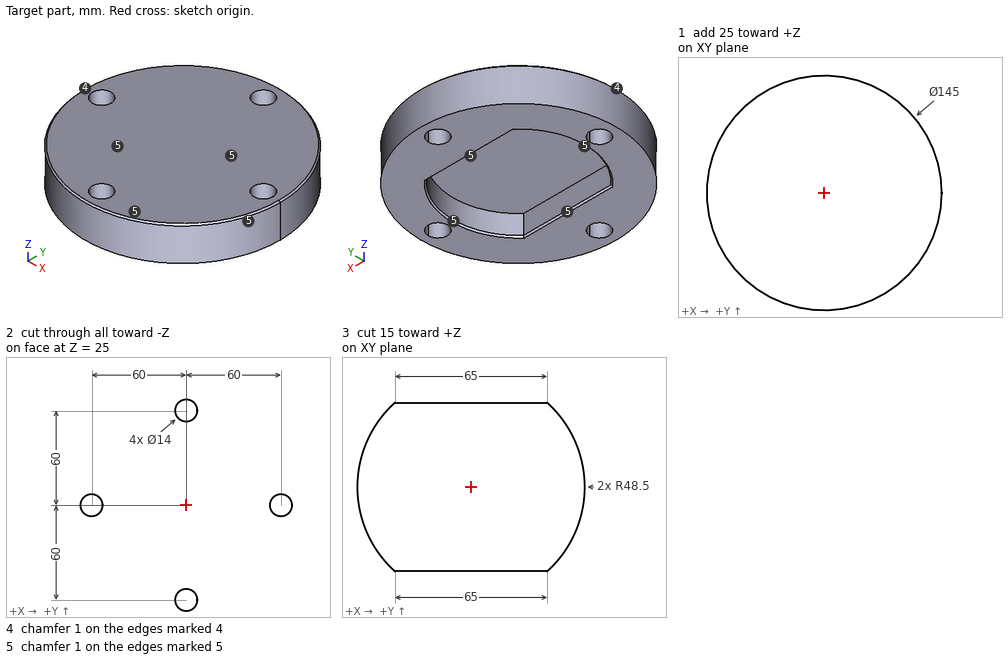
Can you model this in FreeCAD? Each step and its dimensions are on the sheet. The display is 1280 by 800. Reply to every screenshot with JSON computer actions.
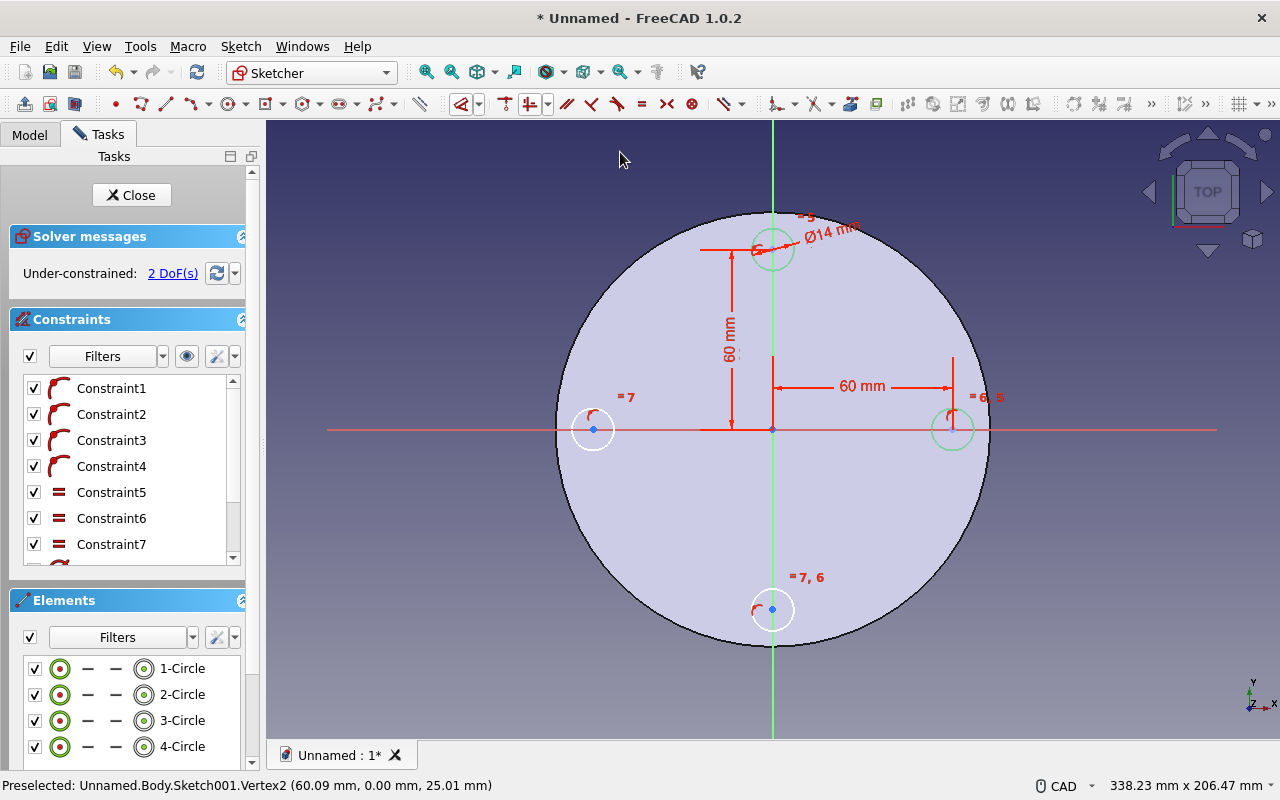
{"action": "left_click", "coordinate": [773, 610]}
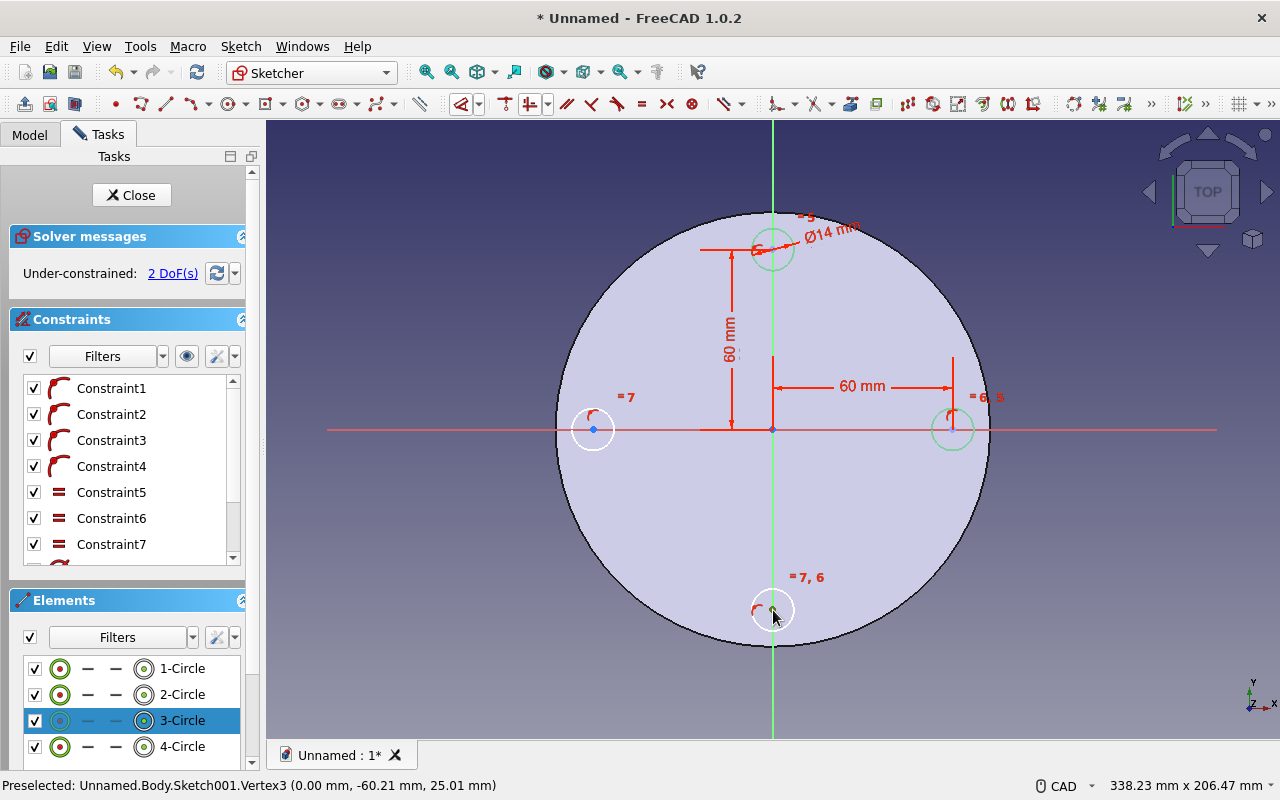
{"action": "key", "text": "i"}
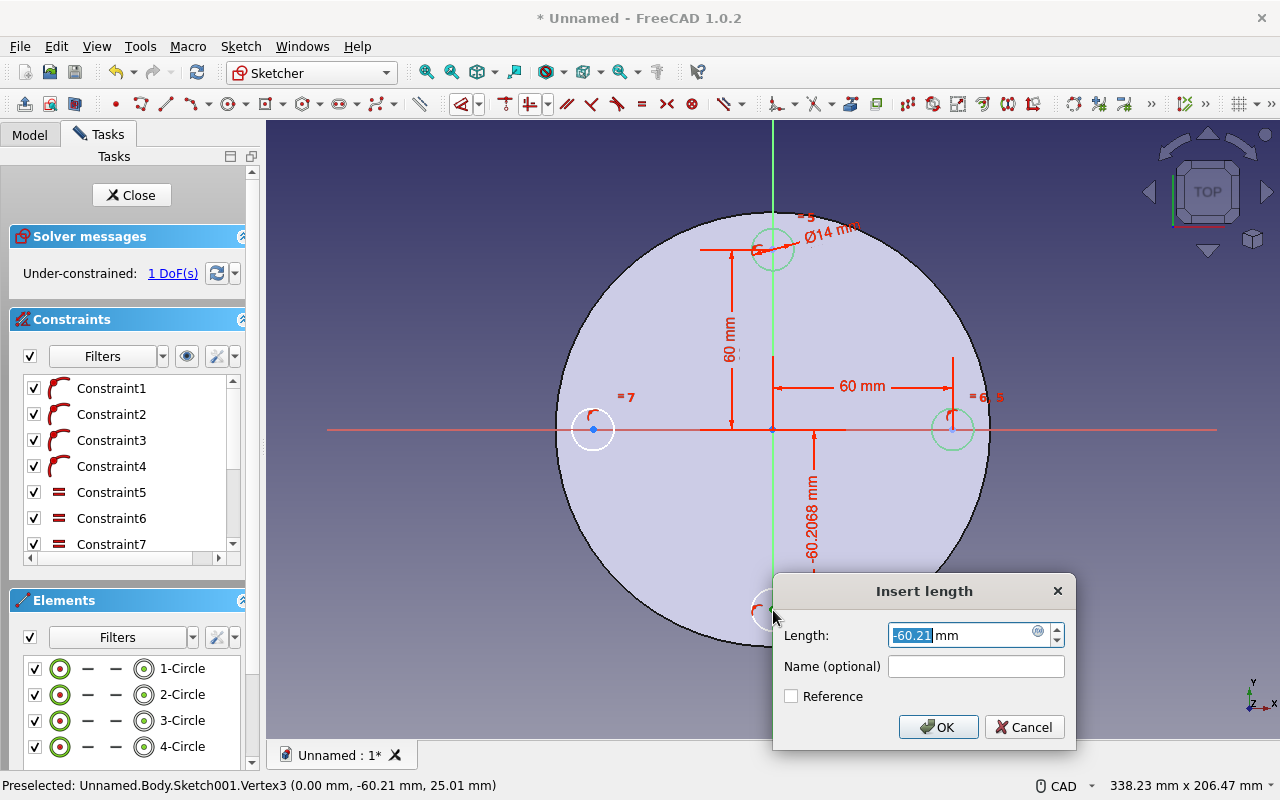
{"action": "type", "text": "-60"}
{"action": "key", "text": "Return"}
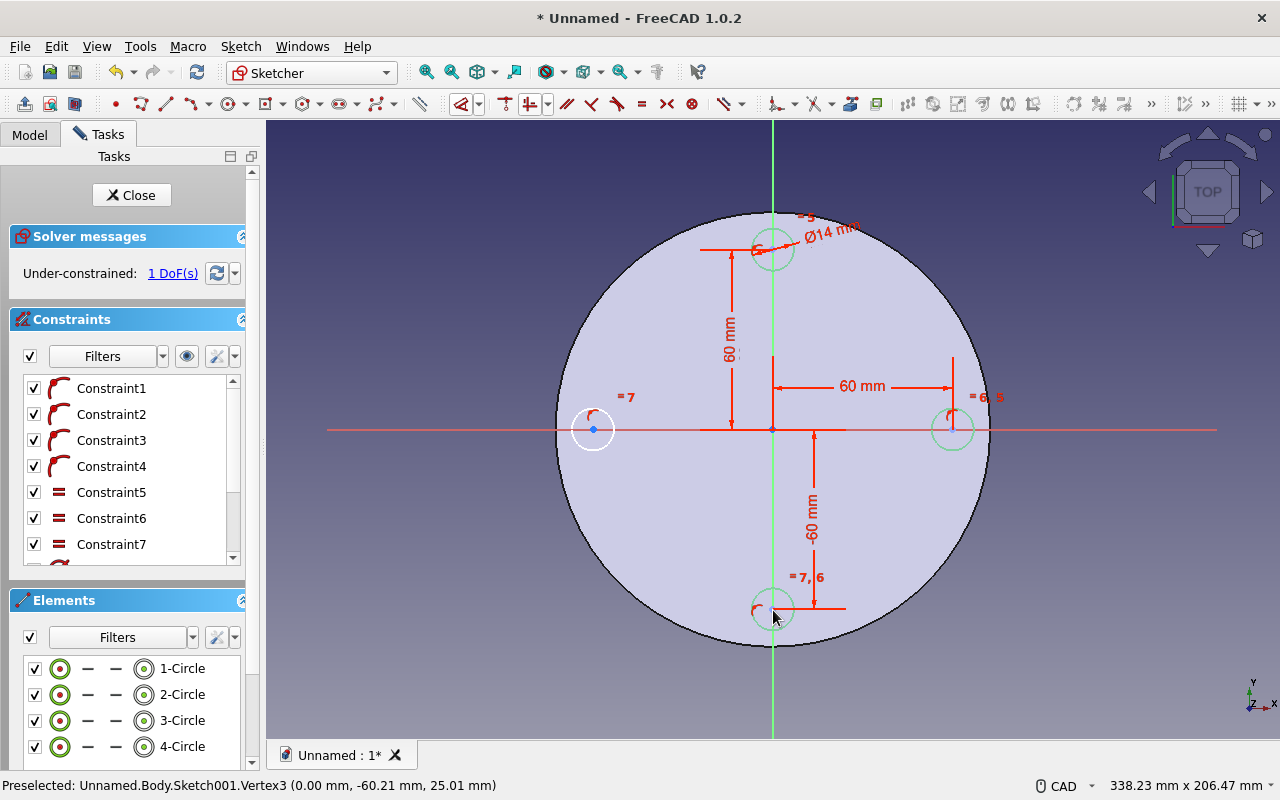
{"action": "left_click", "coordinate": [593, 430]}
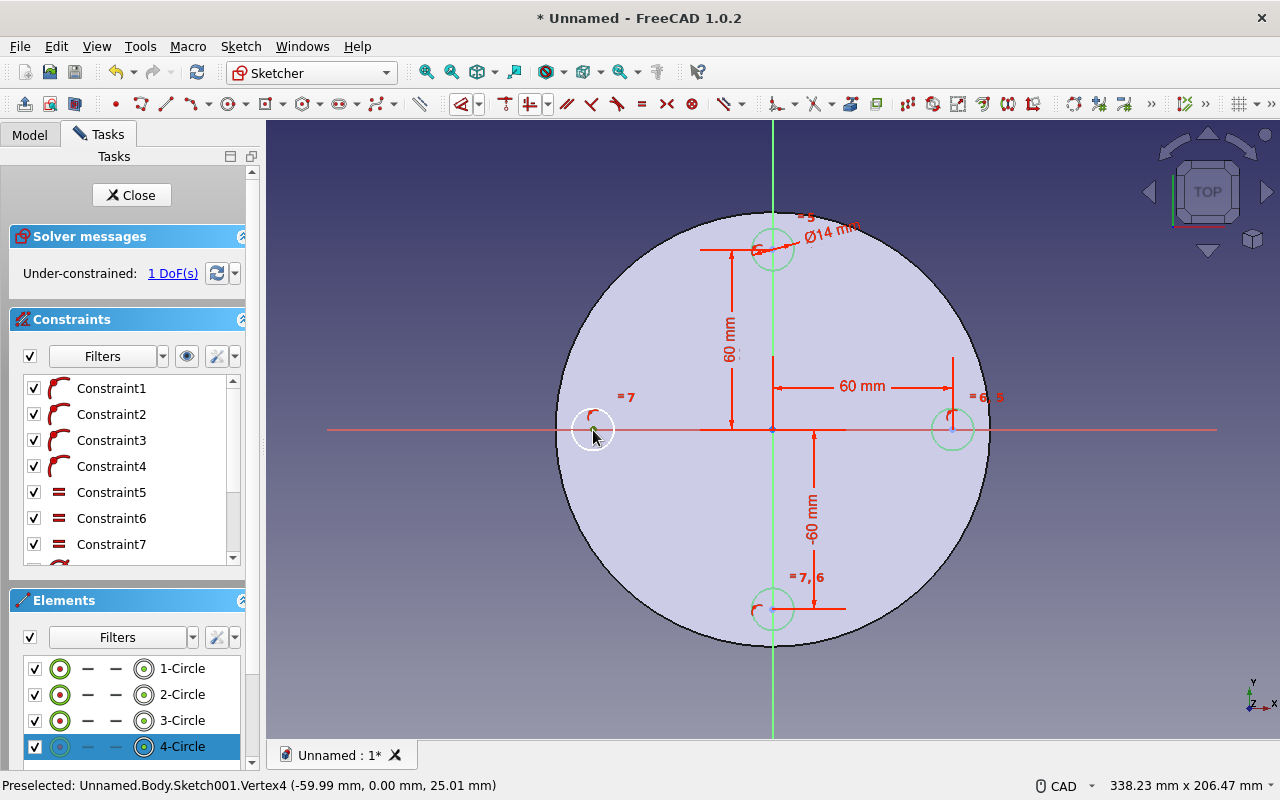
{"action": "left_click", "coordinate": [478, 104]}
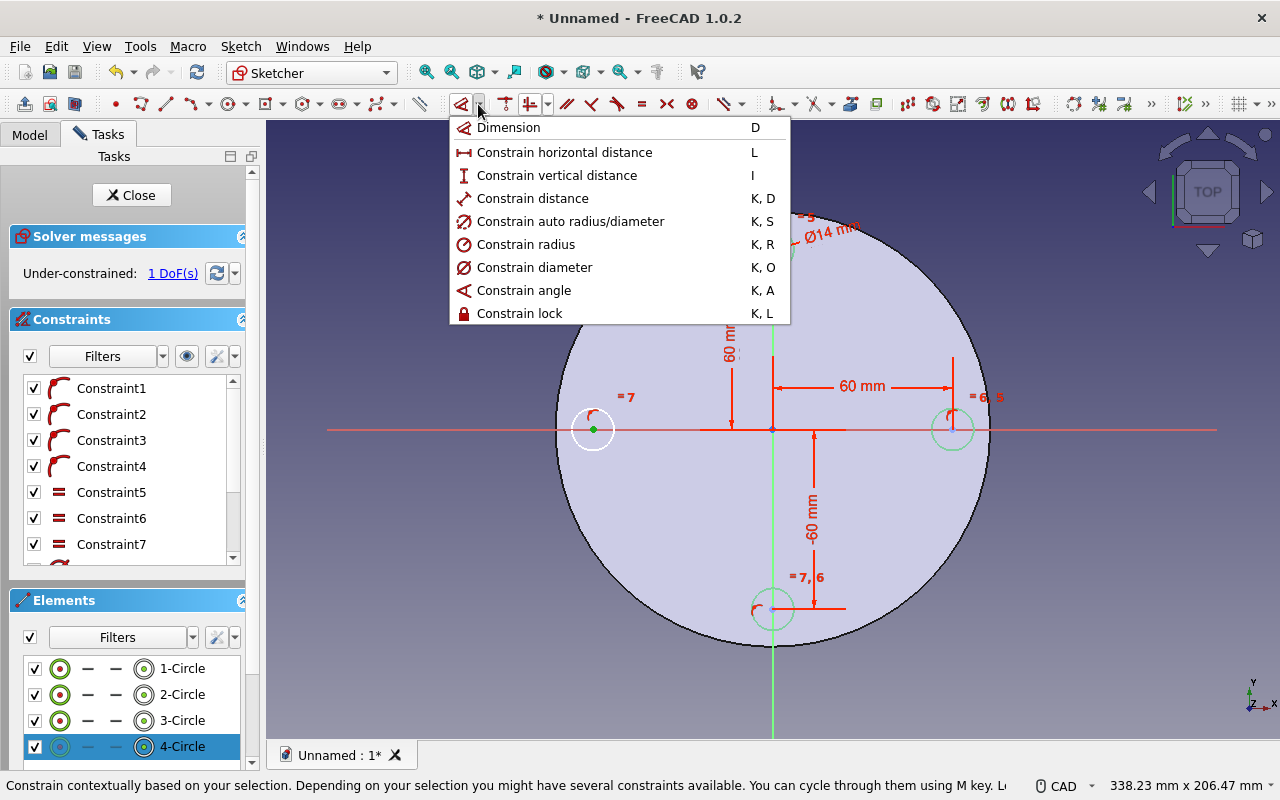
{"action": "left_click", "coordinate": [620, 152]}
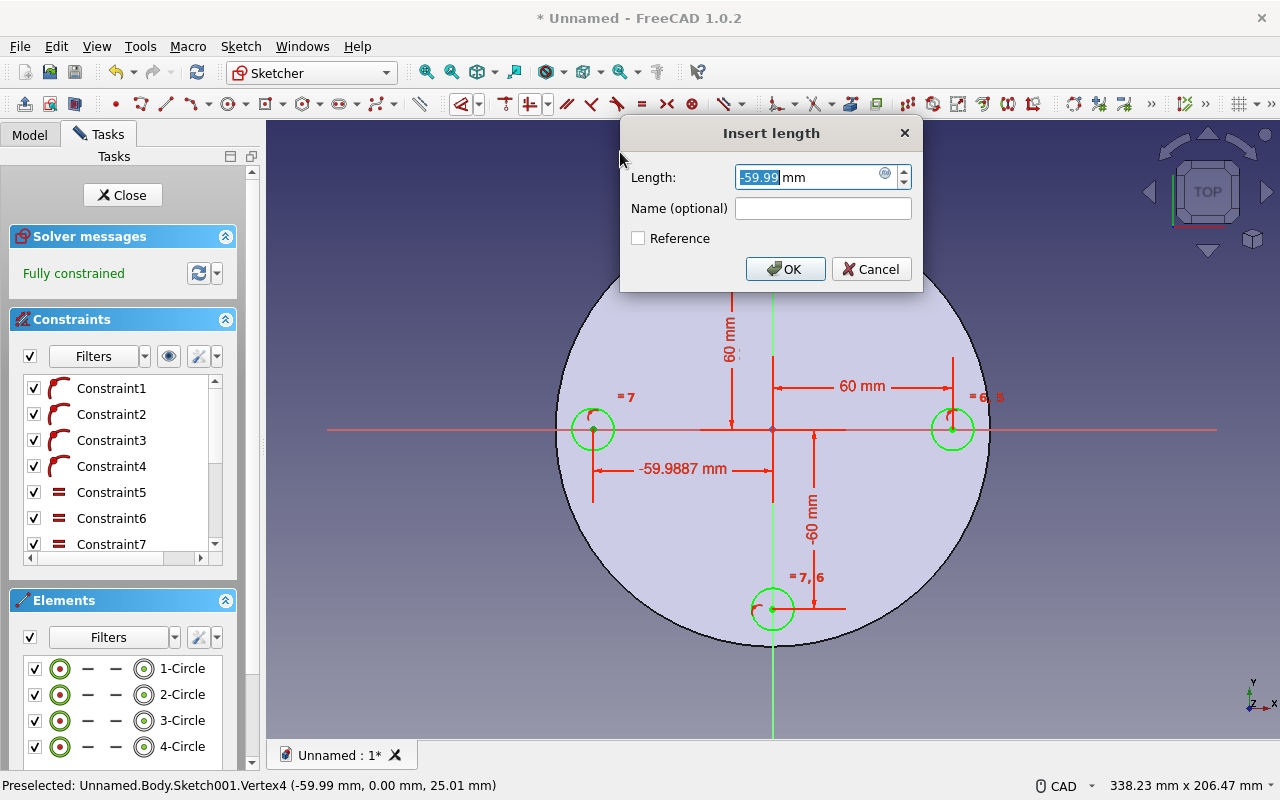
{"action": "type", "text": "-60"}
{"action": "key", "text": "Return"}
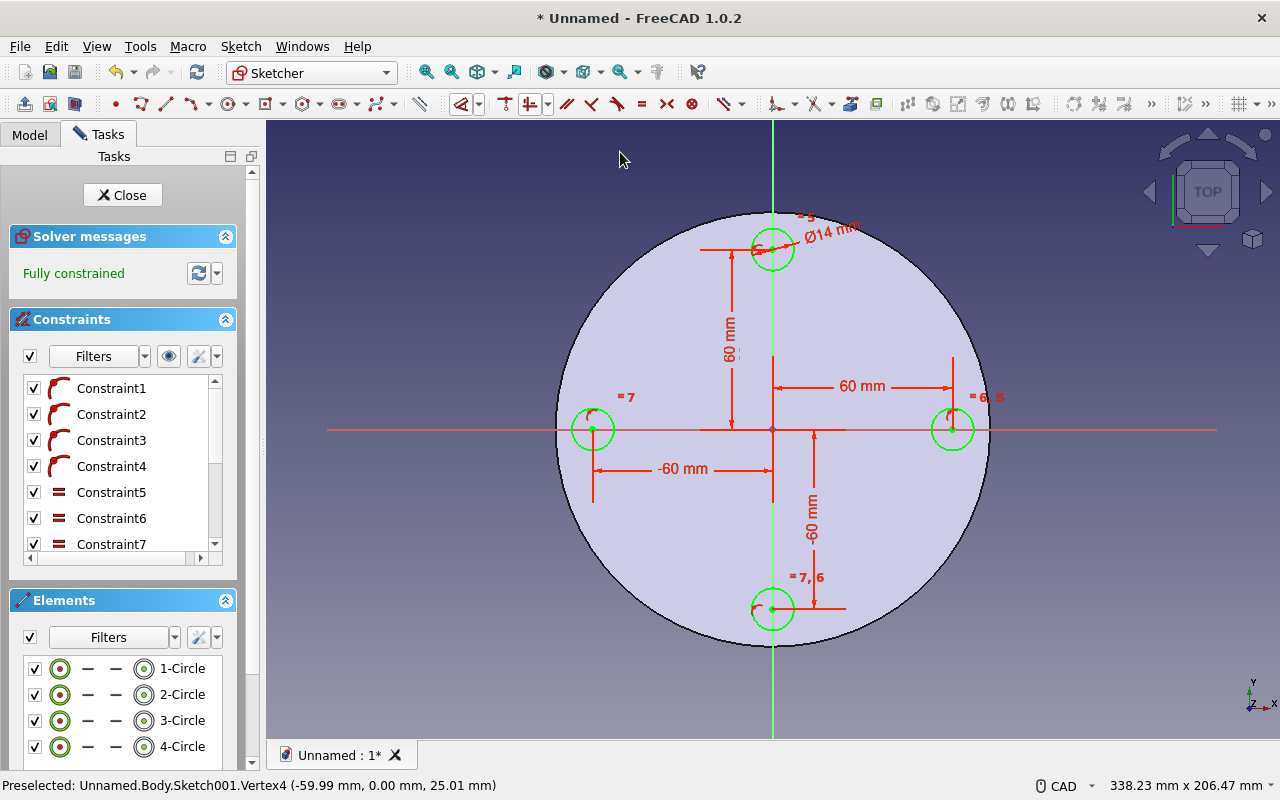
{"action": "left_click", "coordinate": [123, 195]}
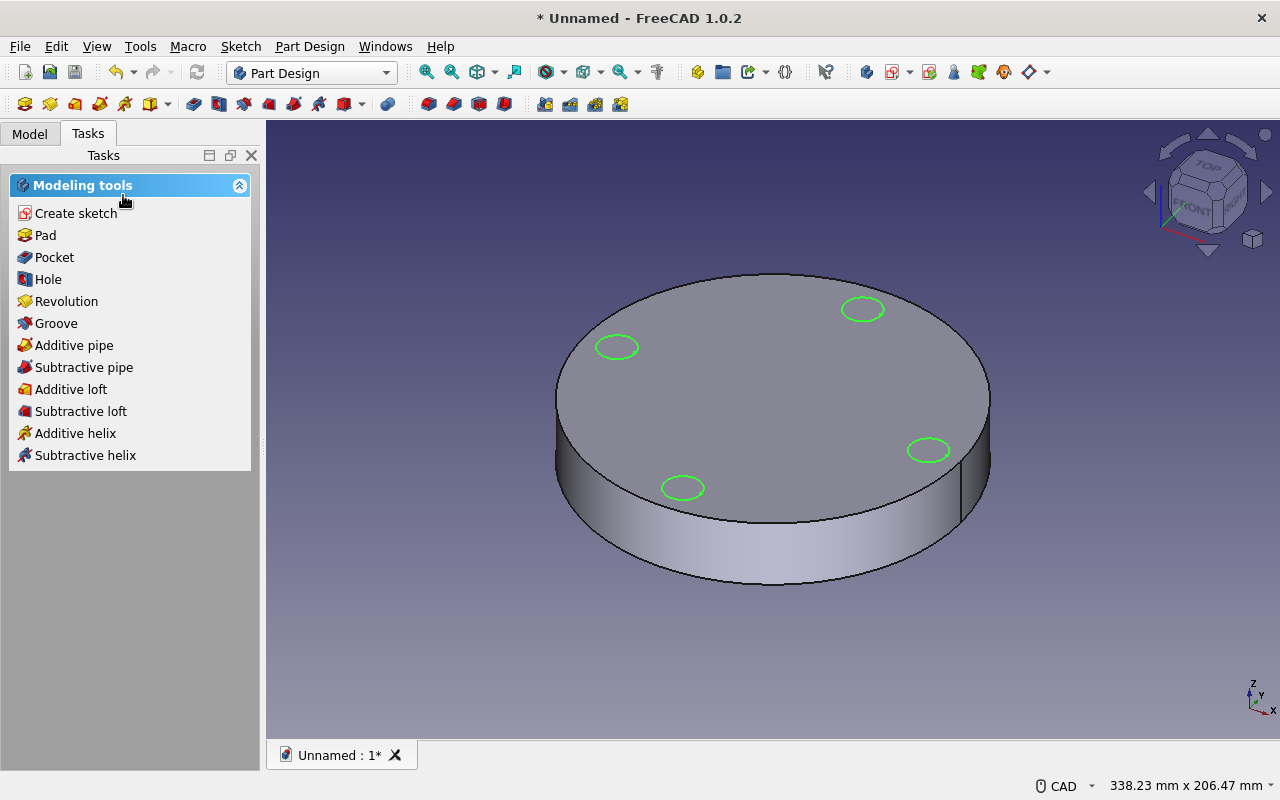
{"action": "left_click", "coordinate": [194, 104]}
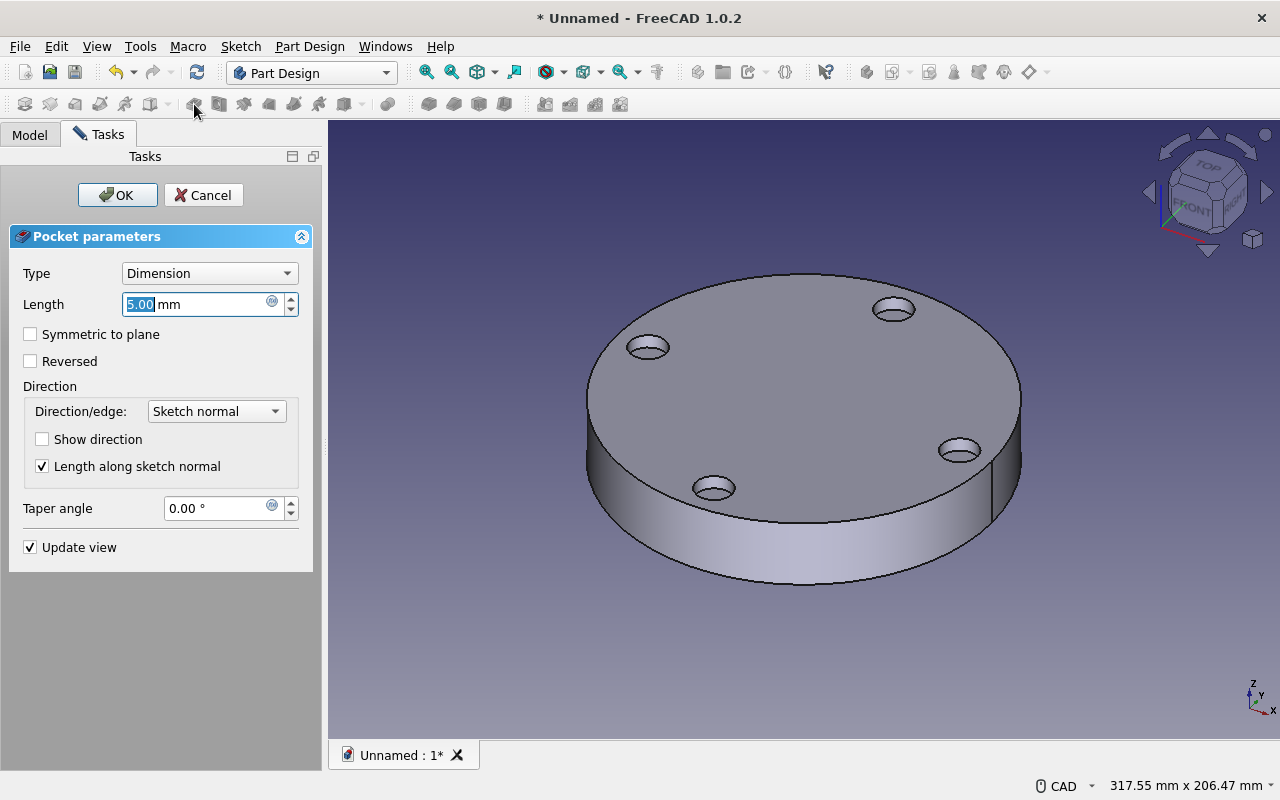
{"action": "left_click", "coordinate": [210, 274]}